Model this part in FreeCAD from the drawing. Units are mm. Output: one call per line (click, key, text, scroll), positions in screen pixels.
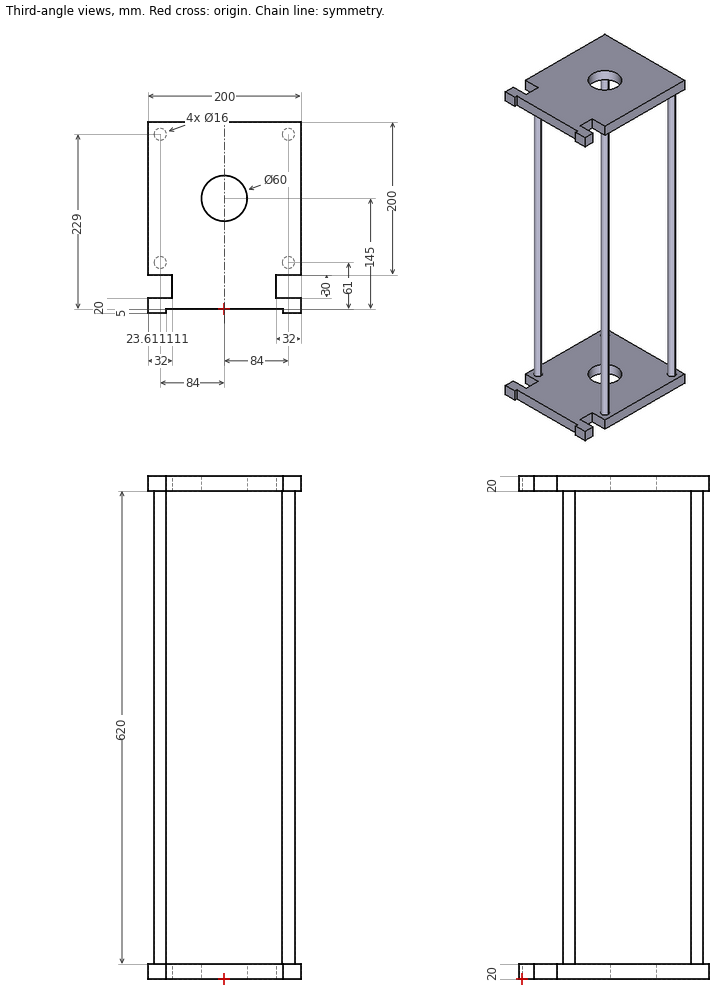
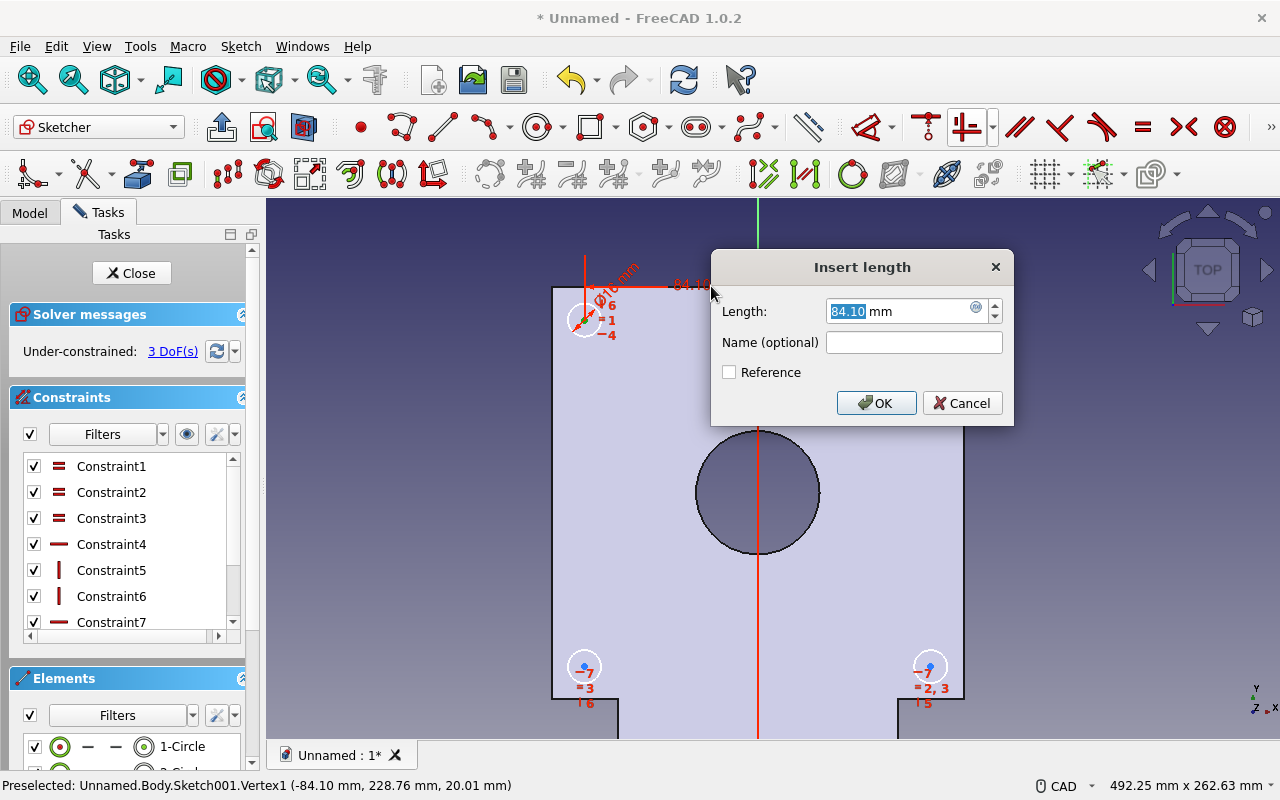
text(84)
key(Return)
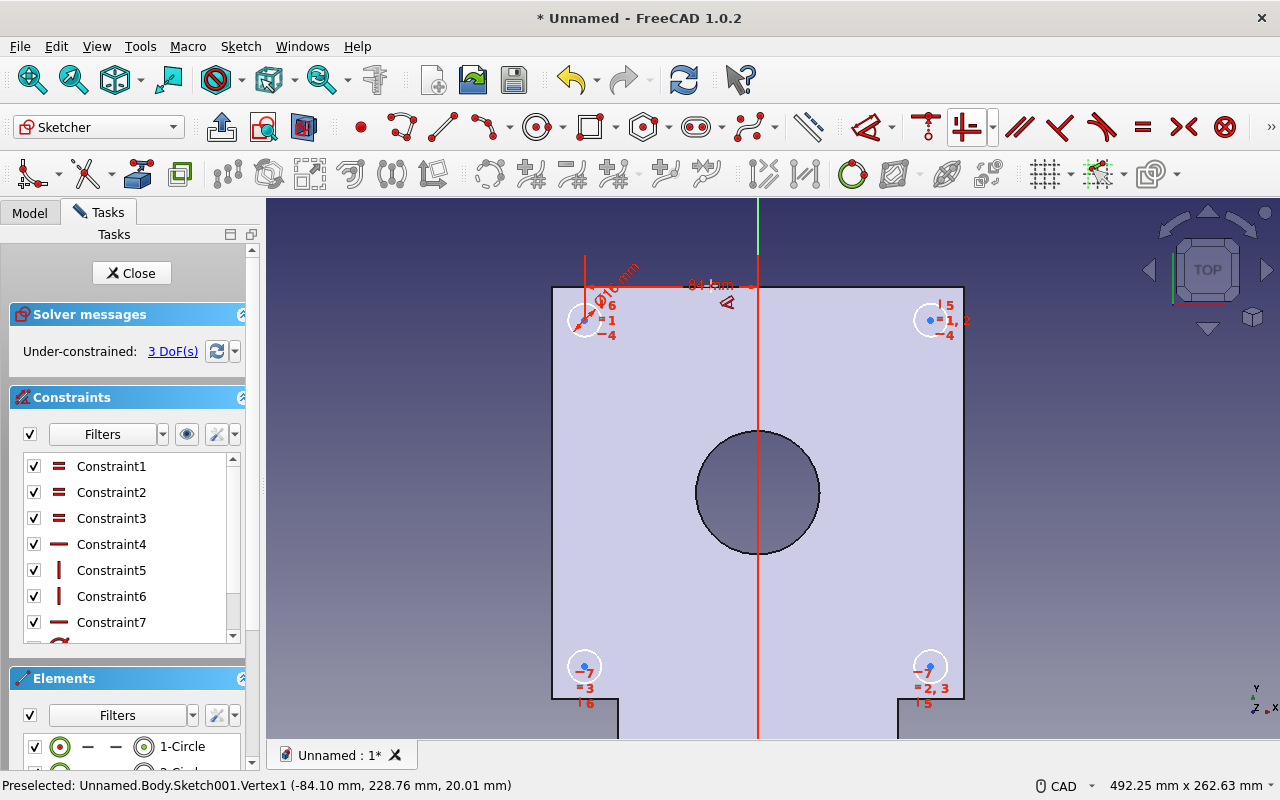
click(931, 320)
click(844, 286)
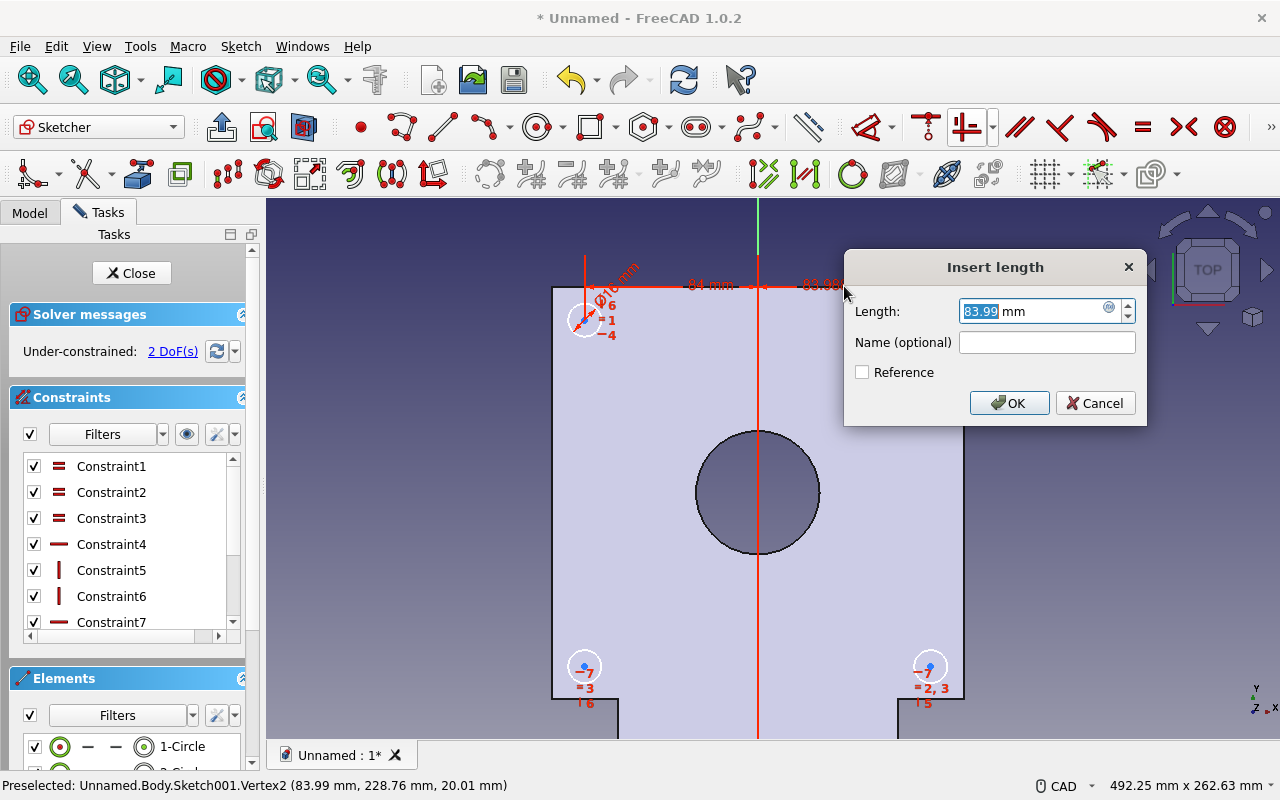
text(84)
key(Return)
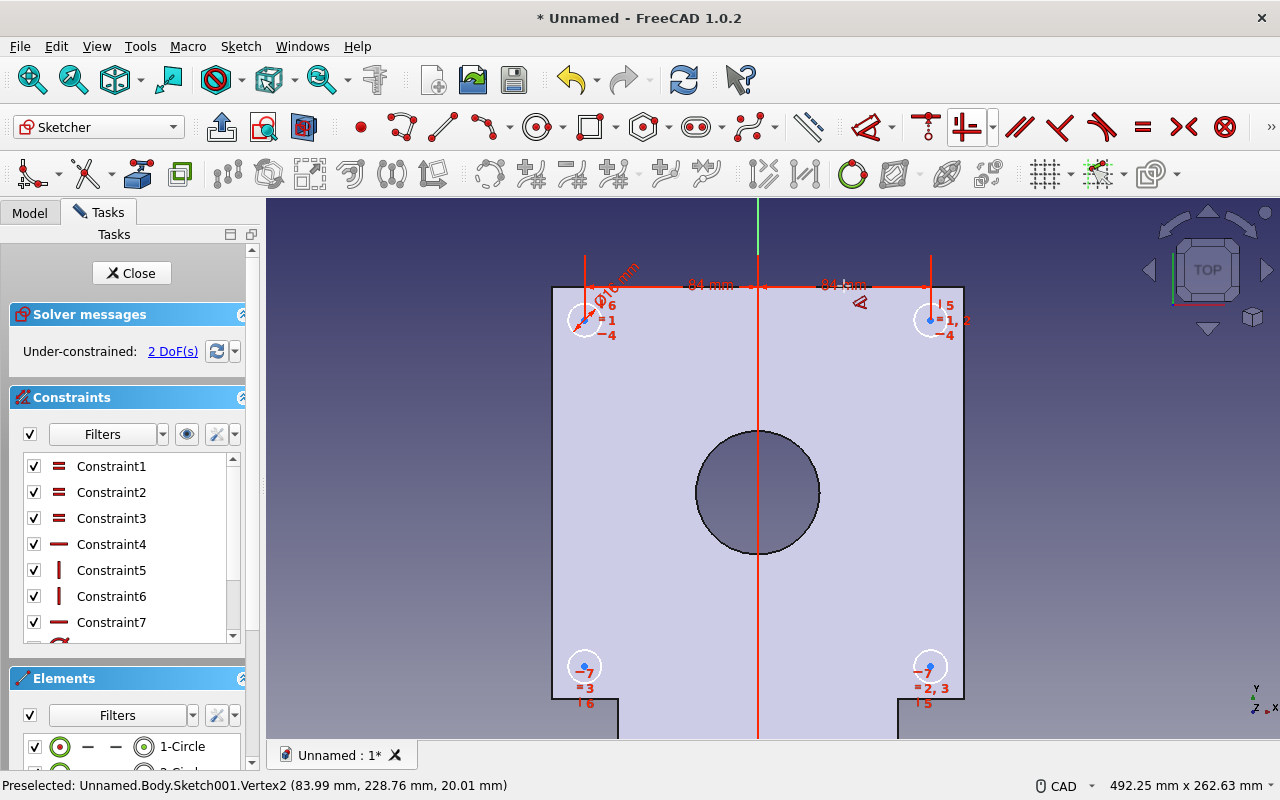
click(931, 667)
click(965, 689)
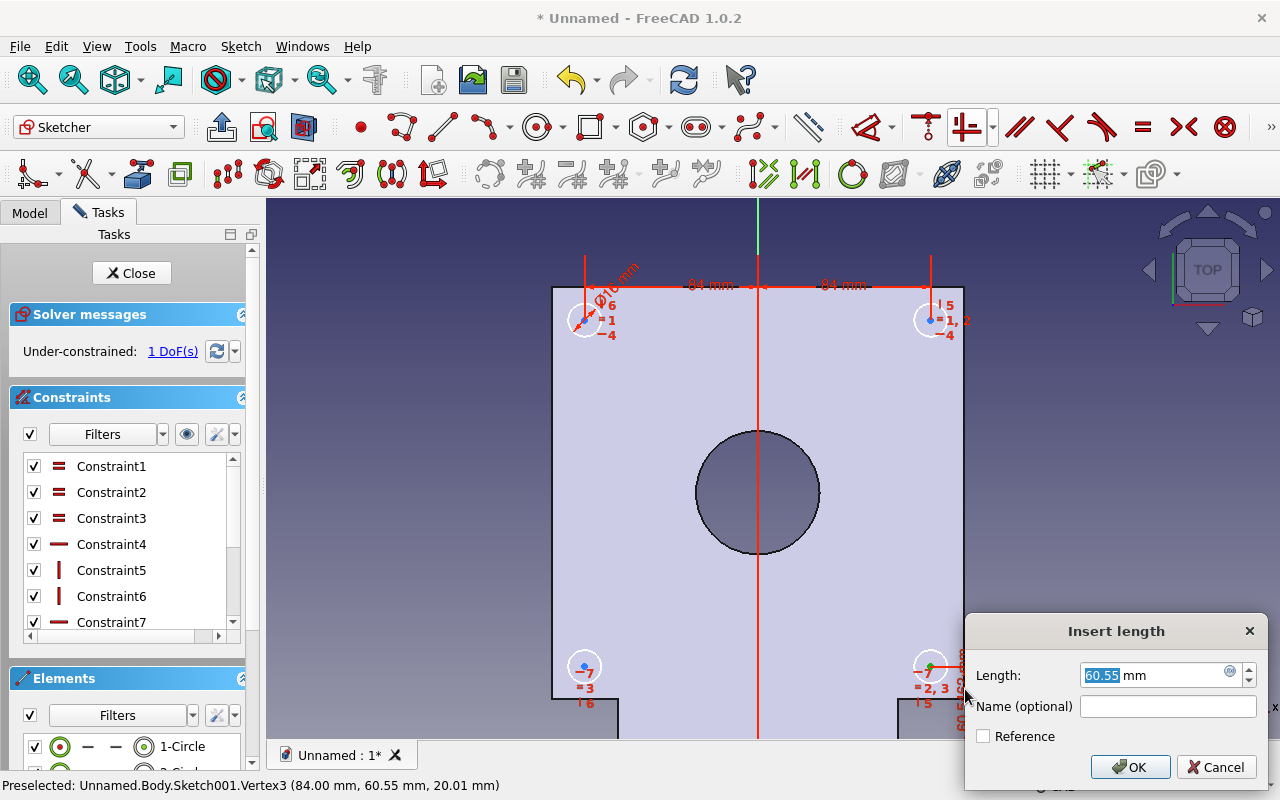
text(61)
key(Return)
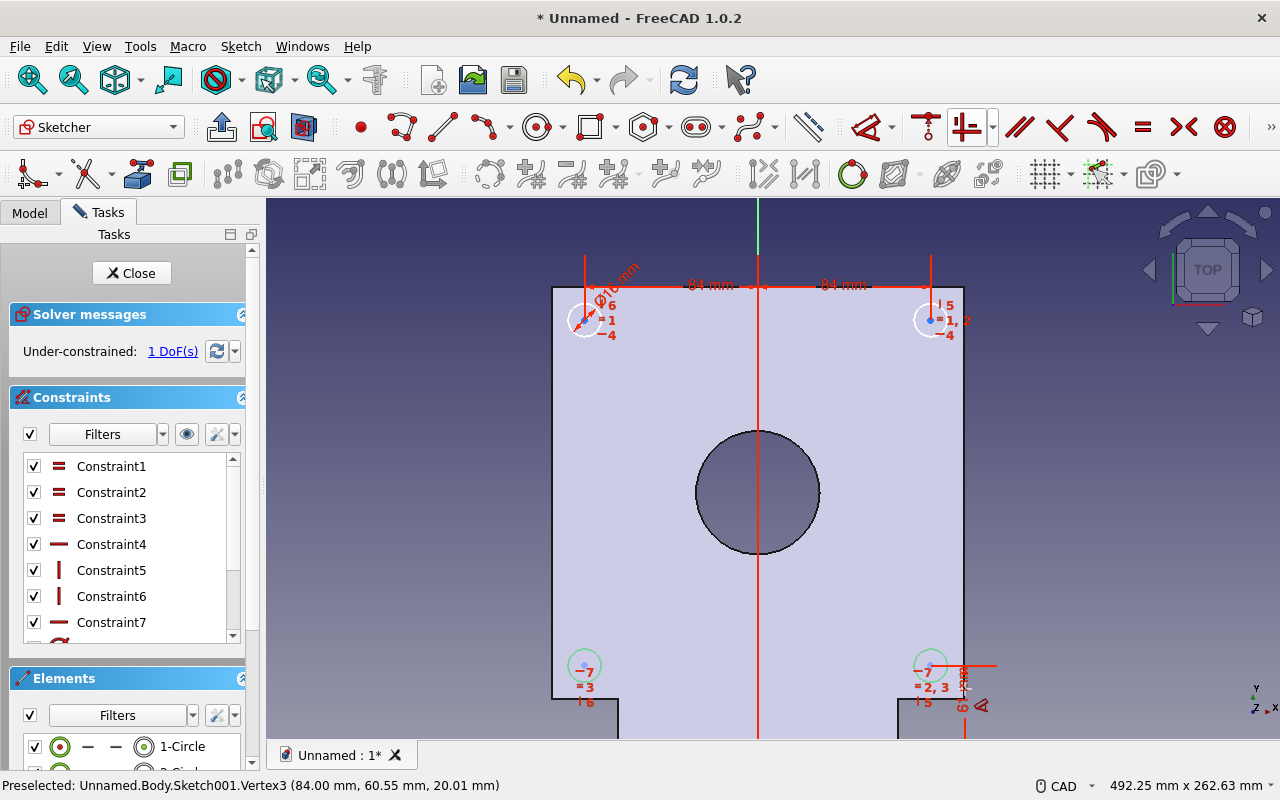
click(585, 320)
click(551, 516)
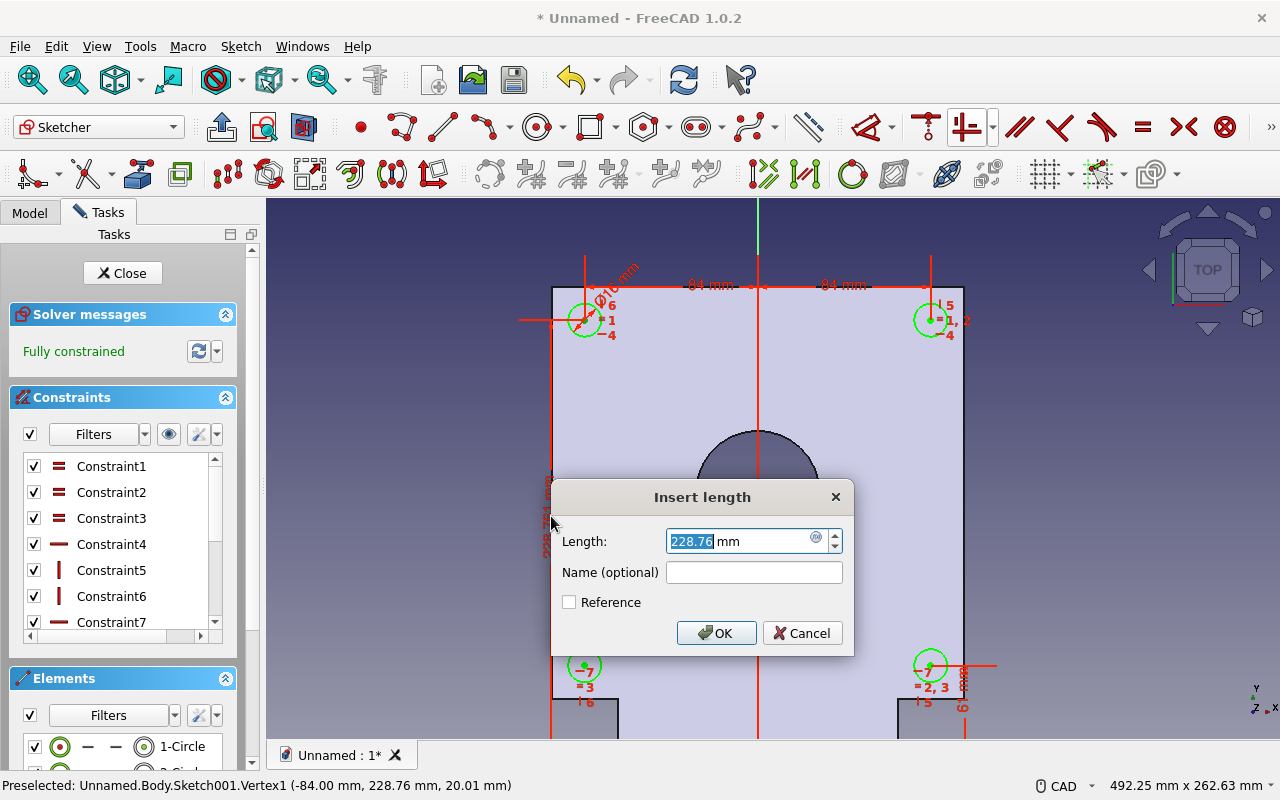
text(229)
key(Return)
key(Escape)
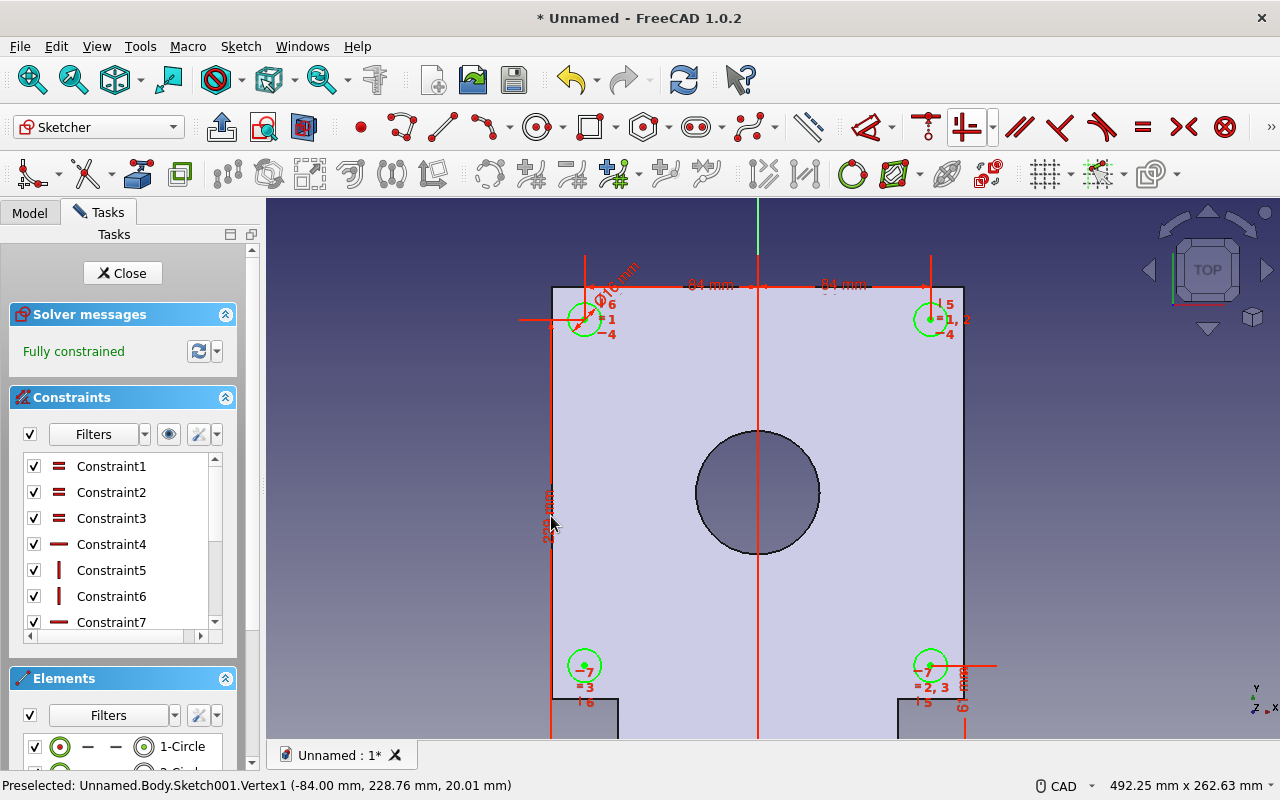
click(123, 273)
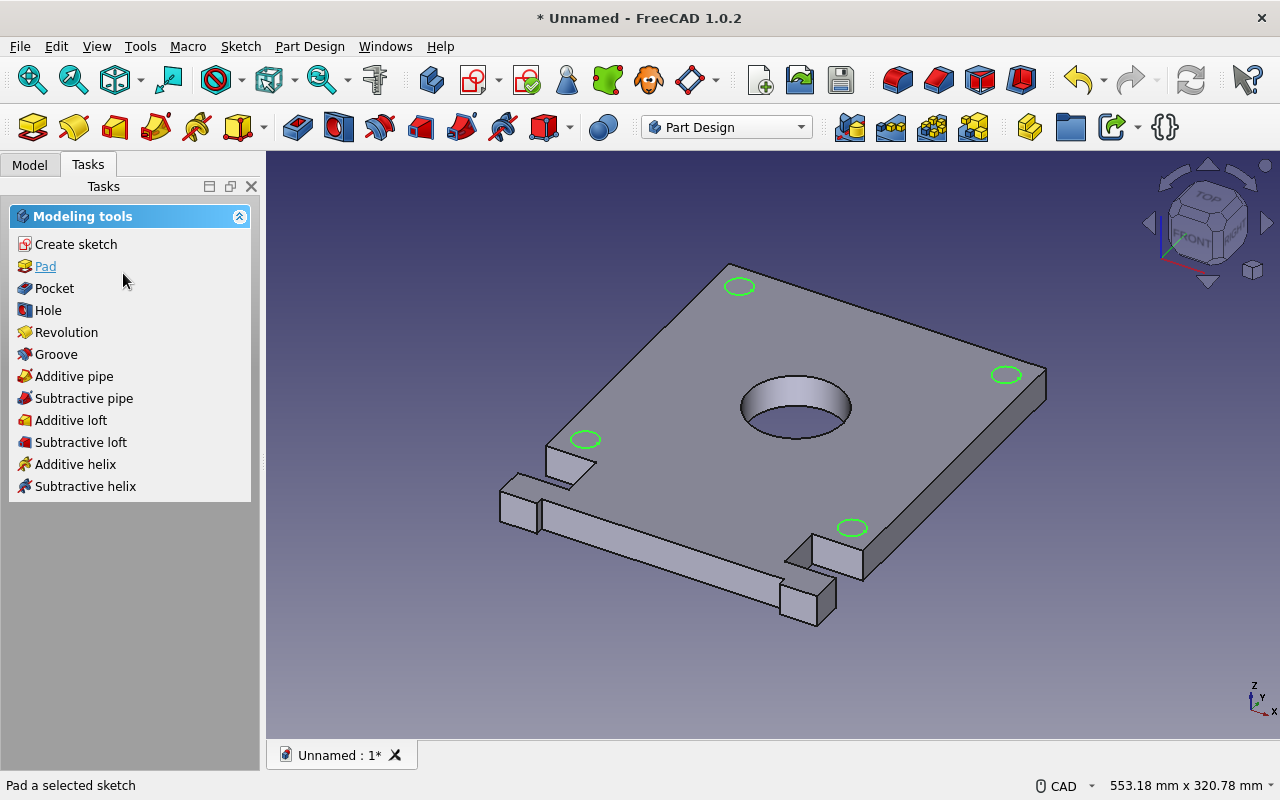
click(33, 128)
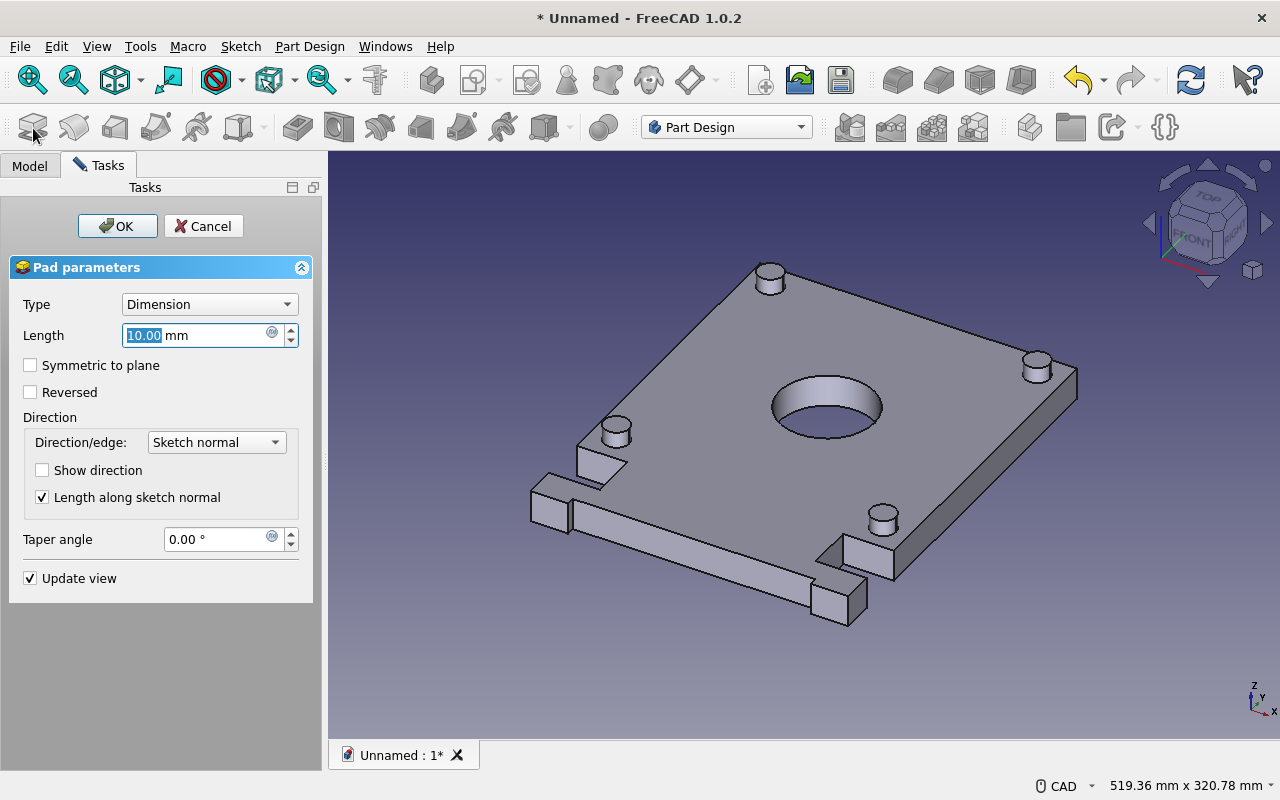
text(620)
key(Tab)